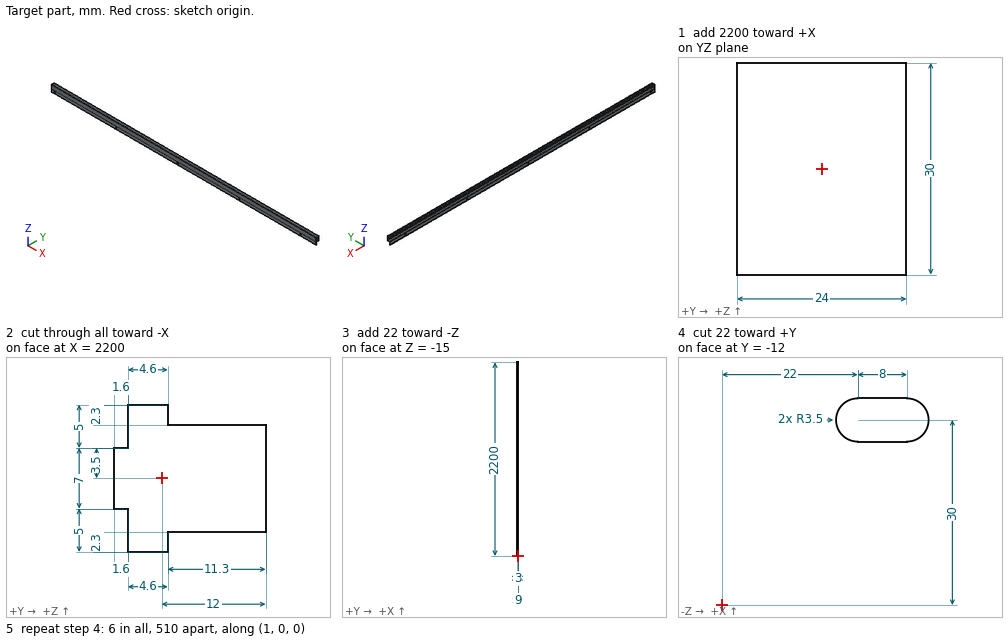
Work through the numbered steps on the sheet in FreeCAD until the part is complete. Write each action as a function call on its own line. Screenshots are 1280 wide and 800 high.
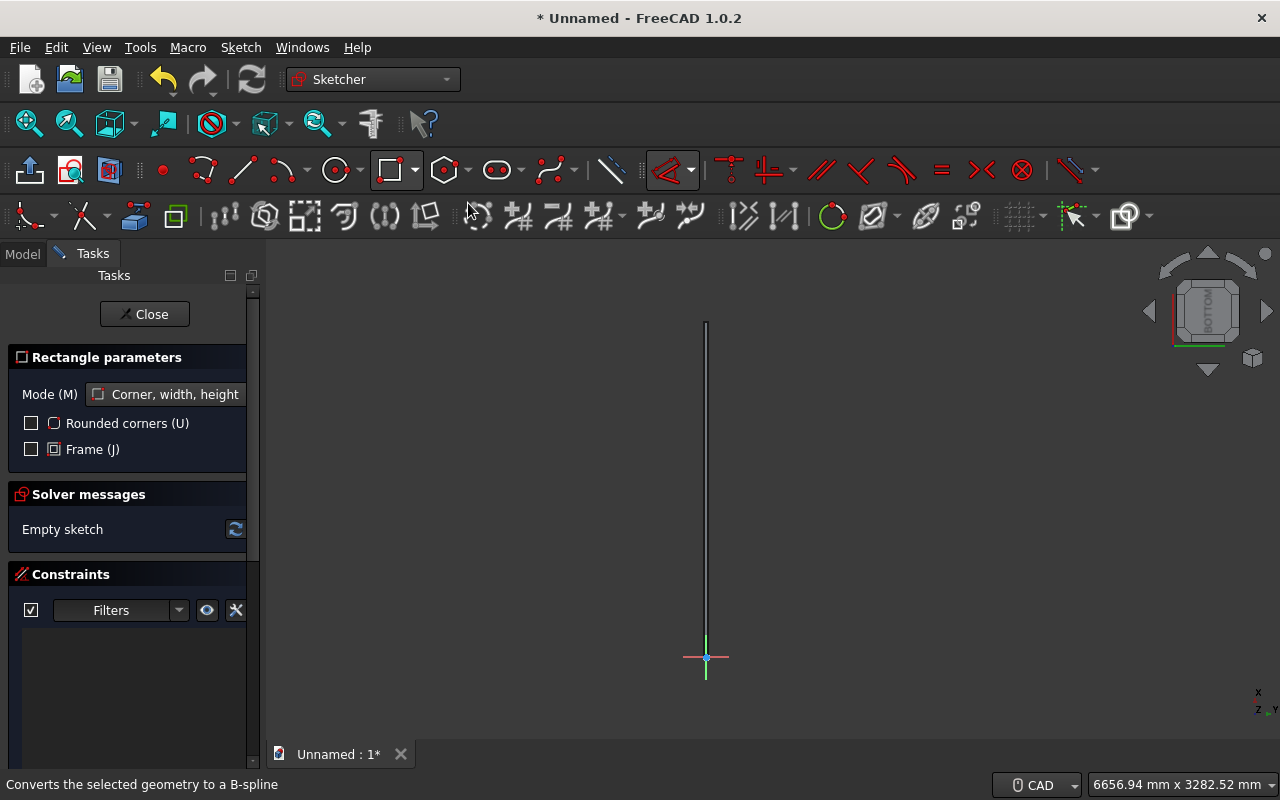
scroll(704, 322, up, 18)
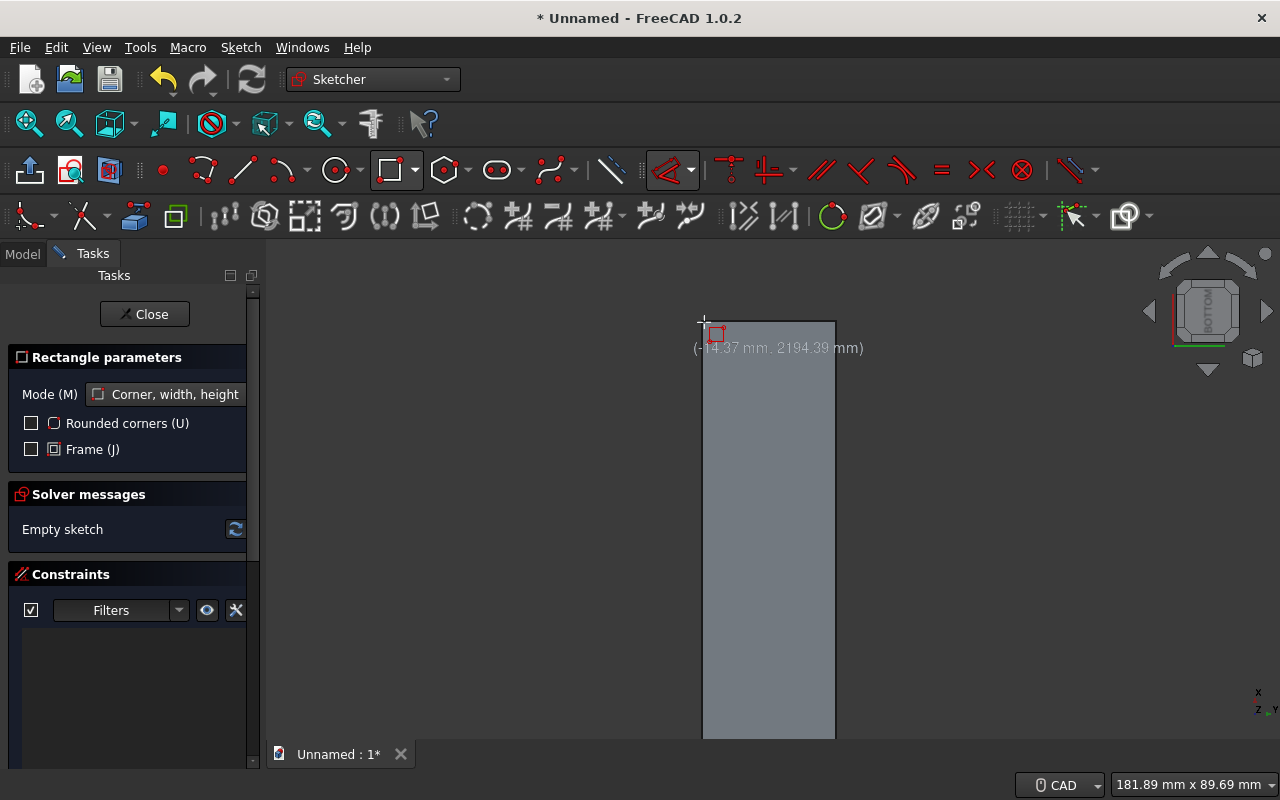
scroll(704, 321, down, 18)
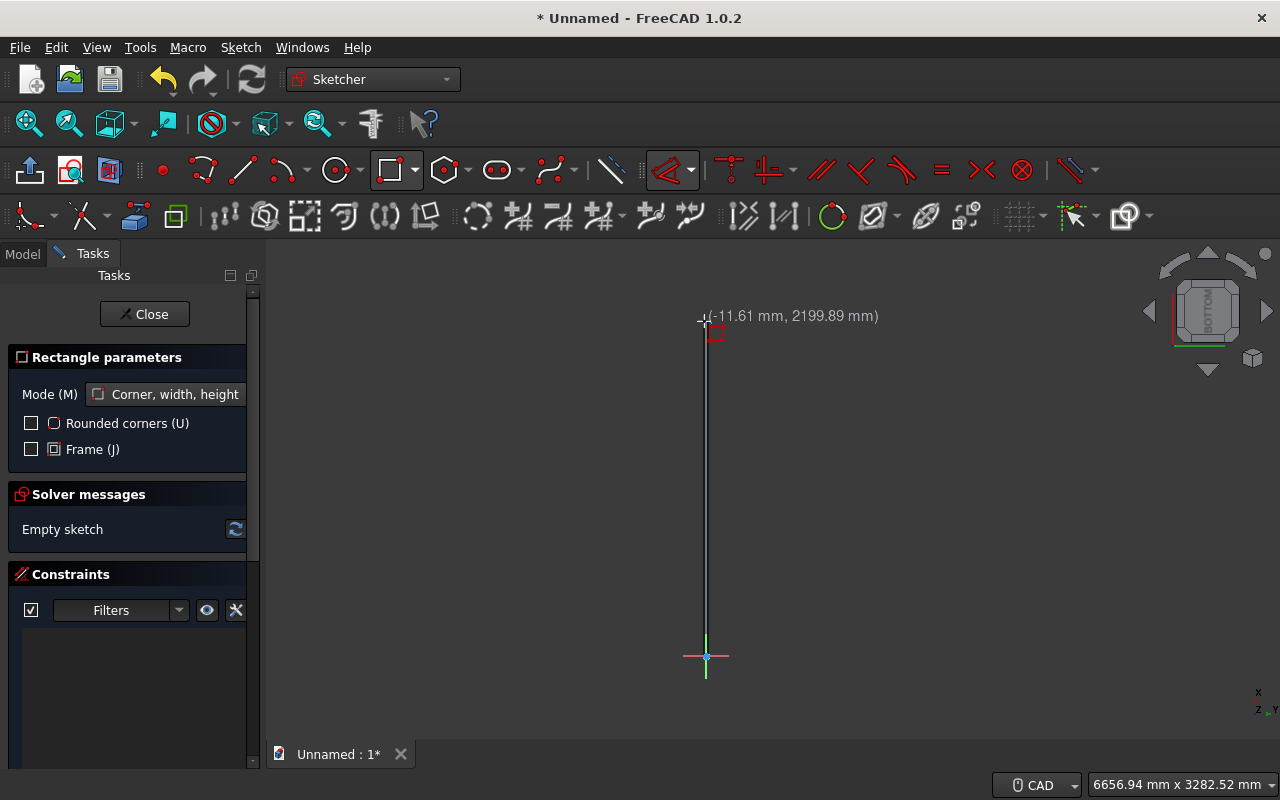
scroll(704, 321, up, 11)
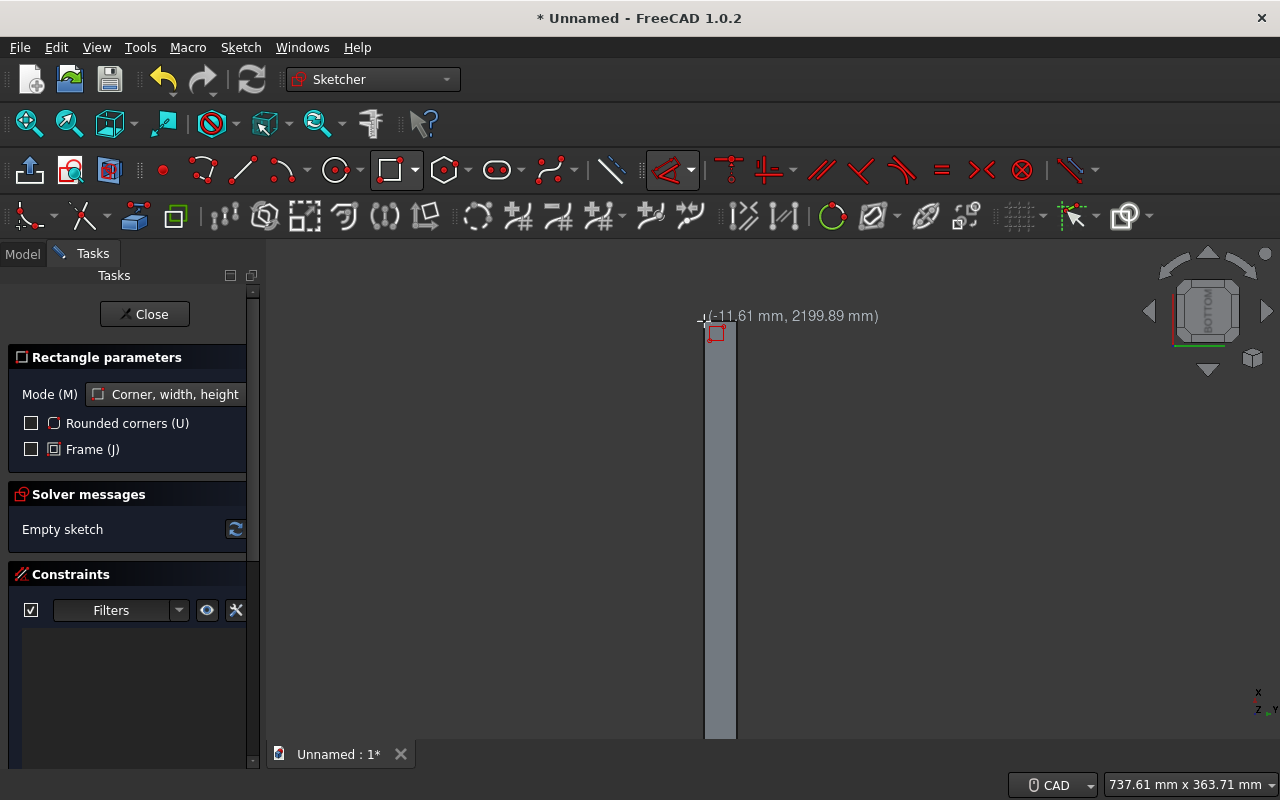
click(704, 321)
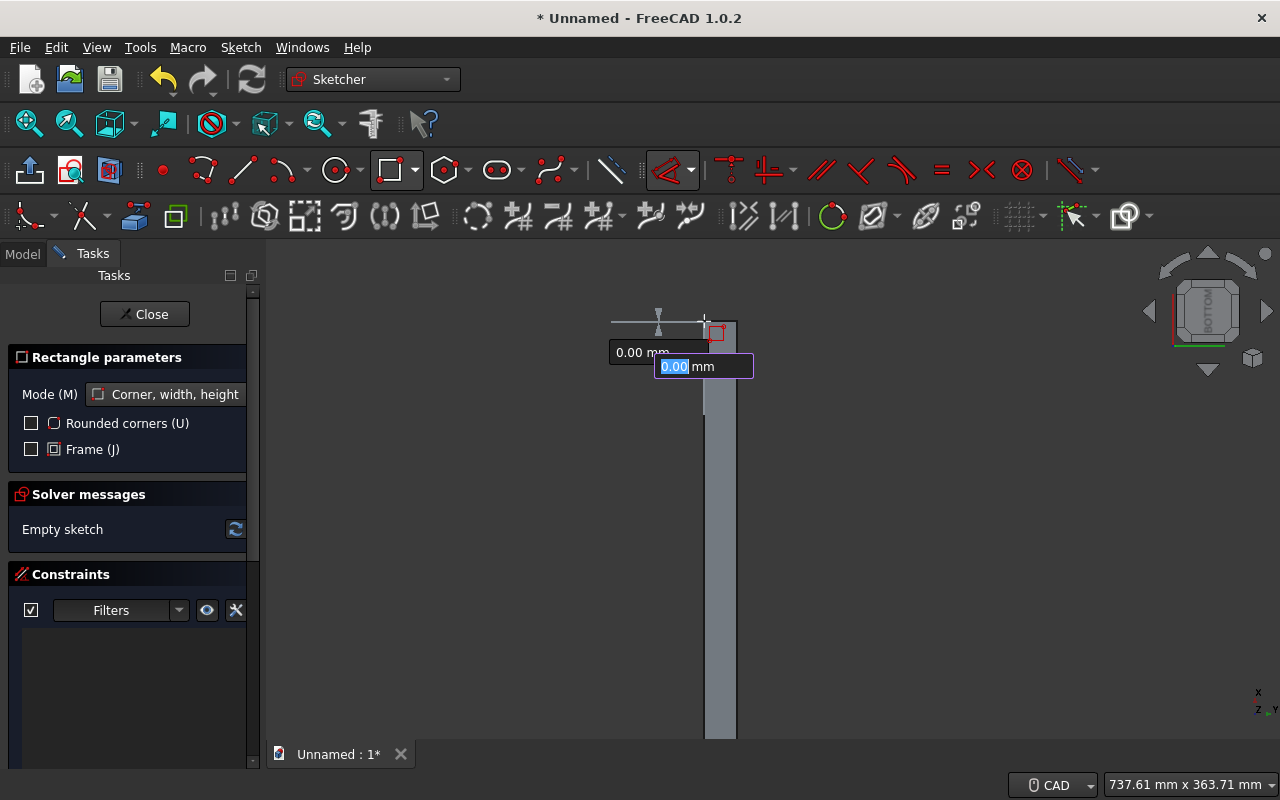
scroll(704, 321, down, 11)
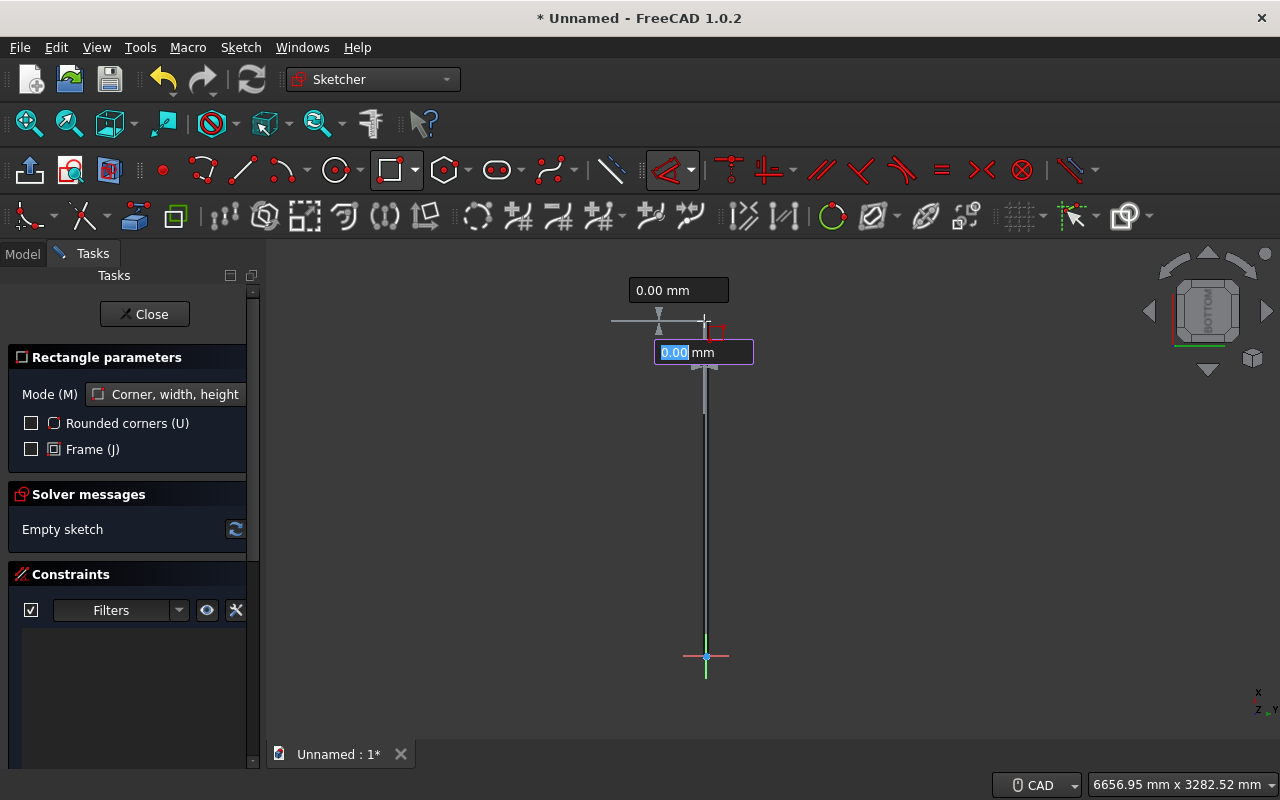
scroll(705, 656, up, 13)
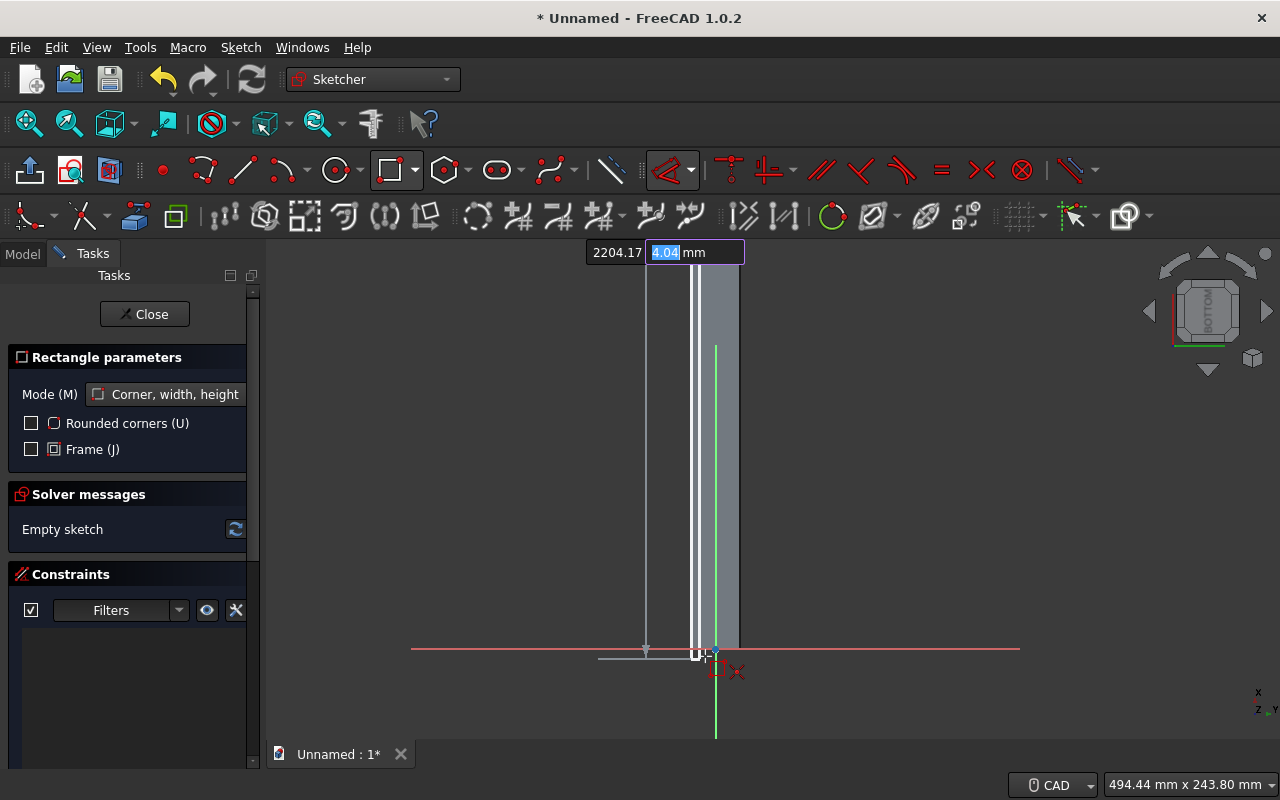
click(697, 649)
key(Escape)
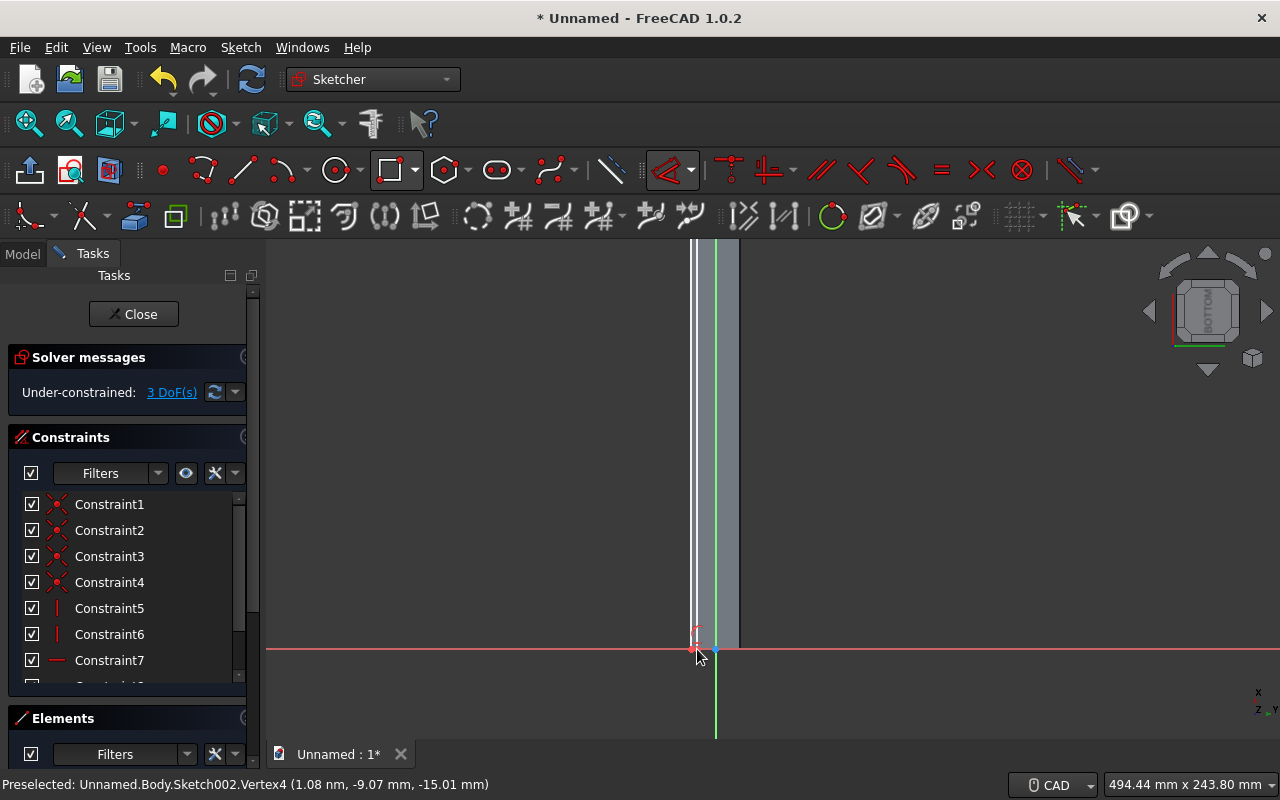
scroll(694, 649, up, 10)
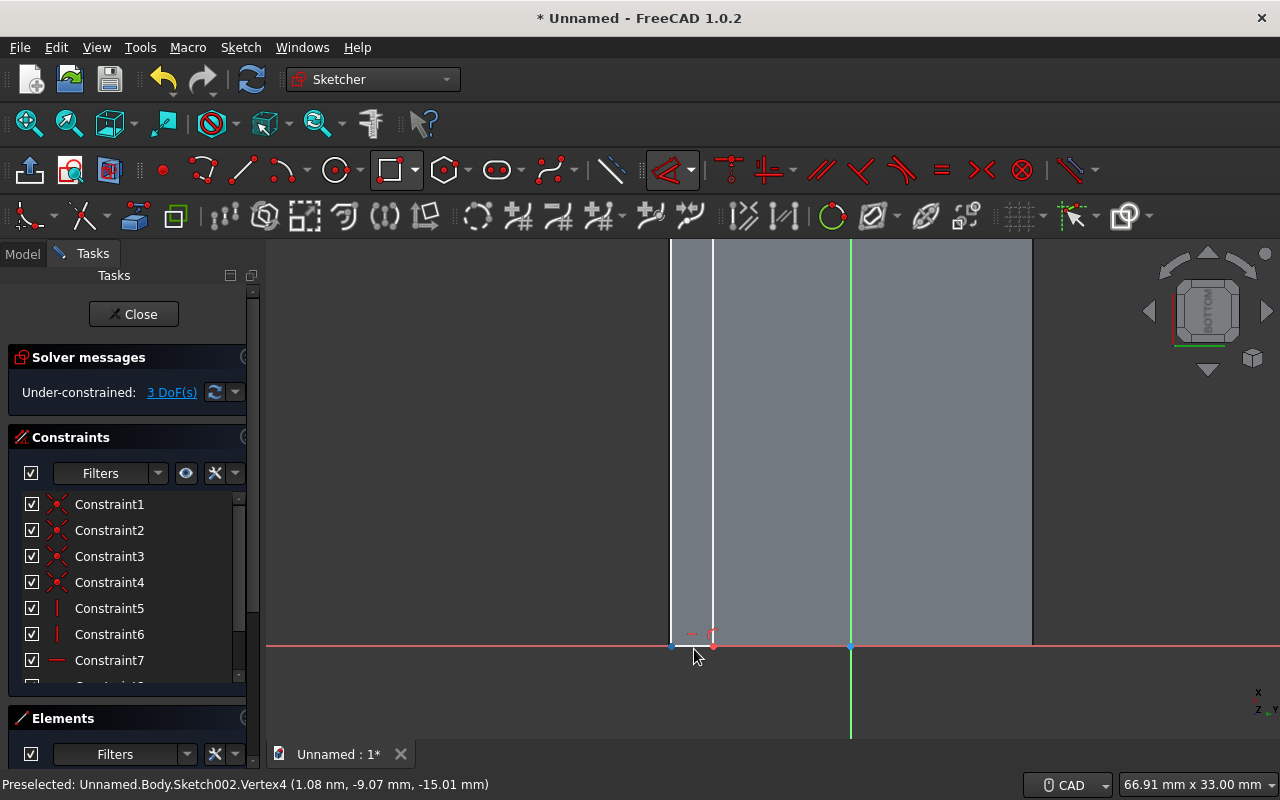
click(692, 646)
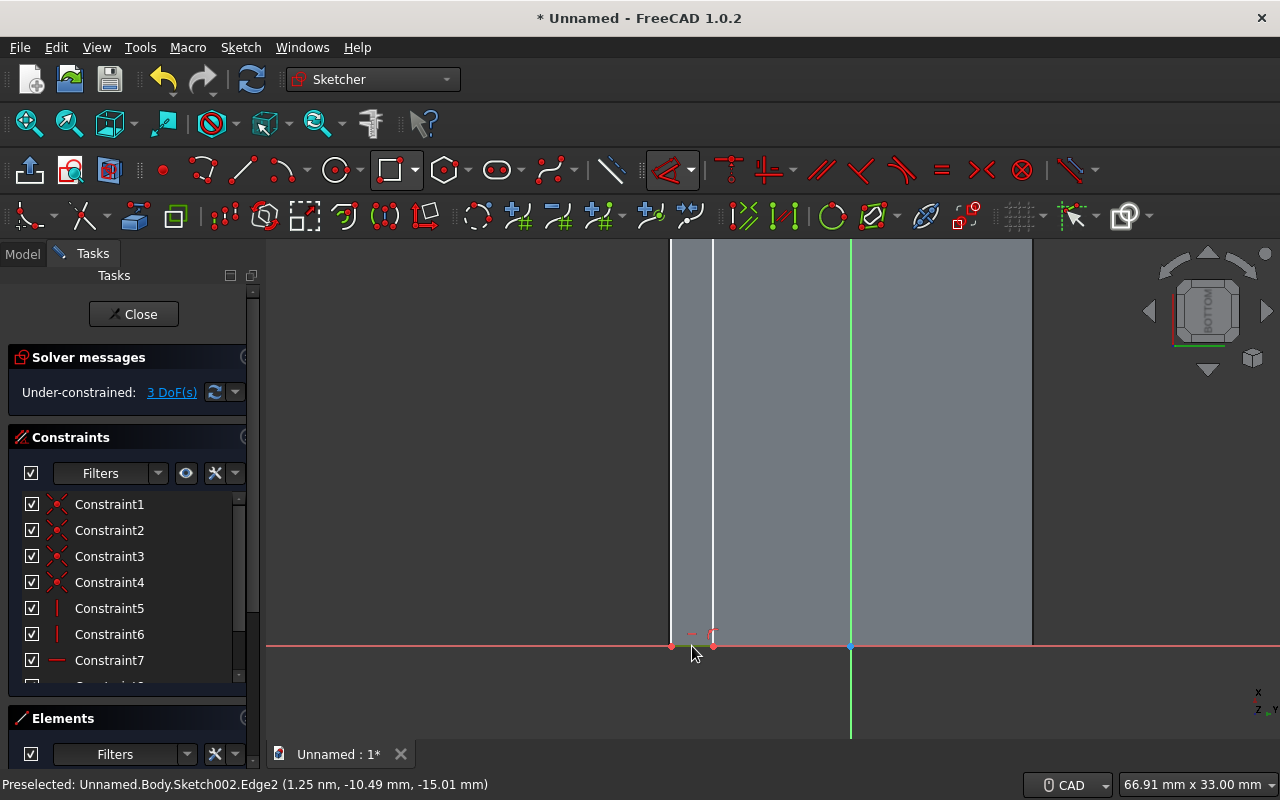
key(l)